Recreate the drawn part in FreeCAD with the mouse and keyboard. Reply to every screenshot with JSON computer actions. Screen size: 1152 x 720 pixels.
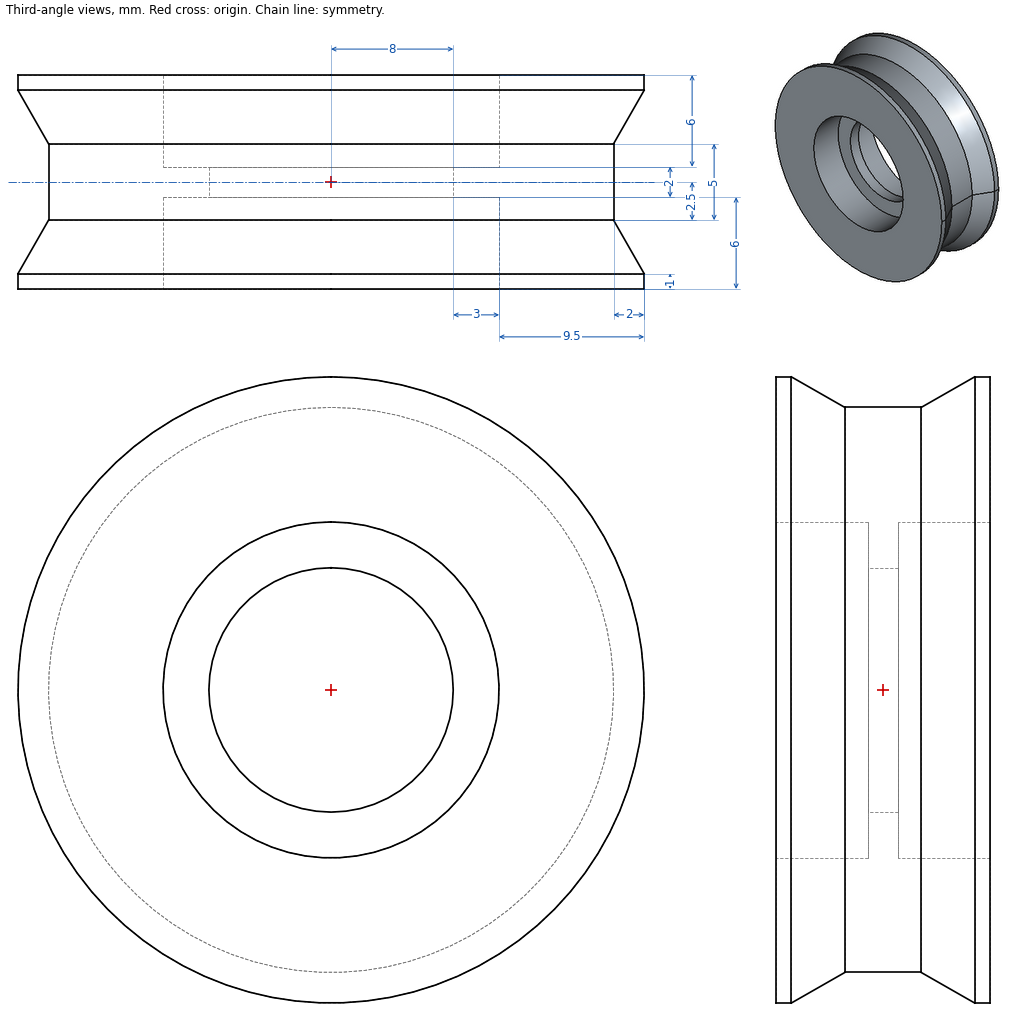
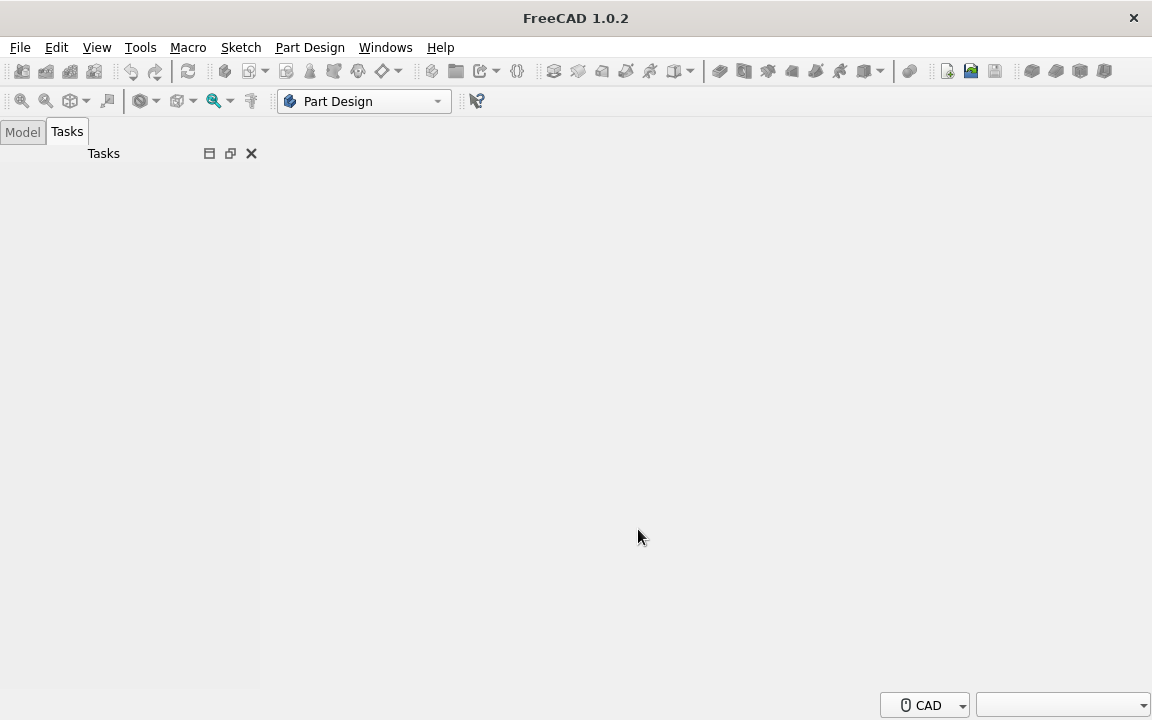
{"action": "left_click", "coordinate": [948, 72]}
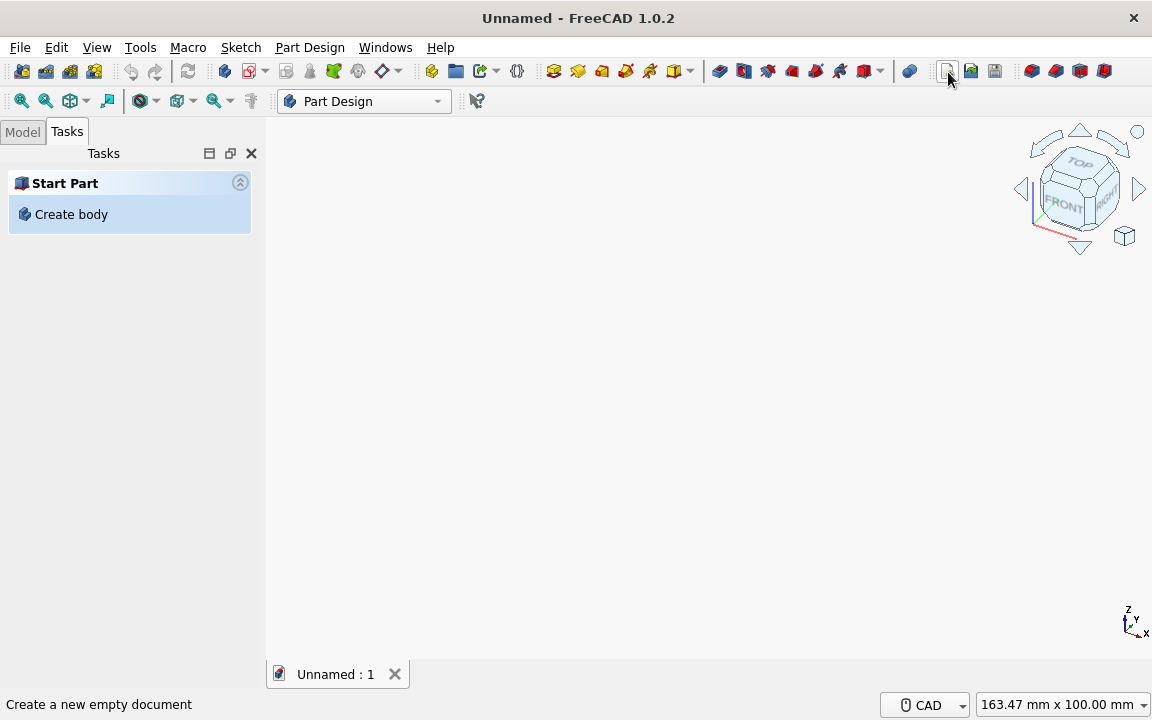
{"action": "left_click", "coordinate": [250, 72]}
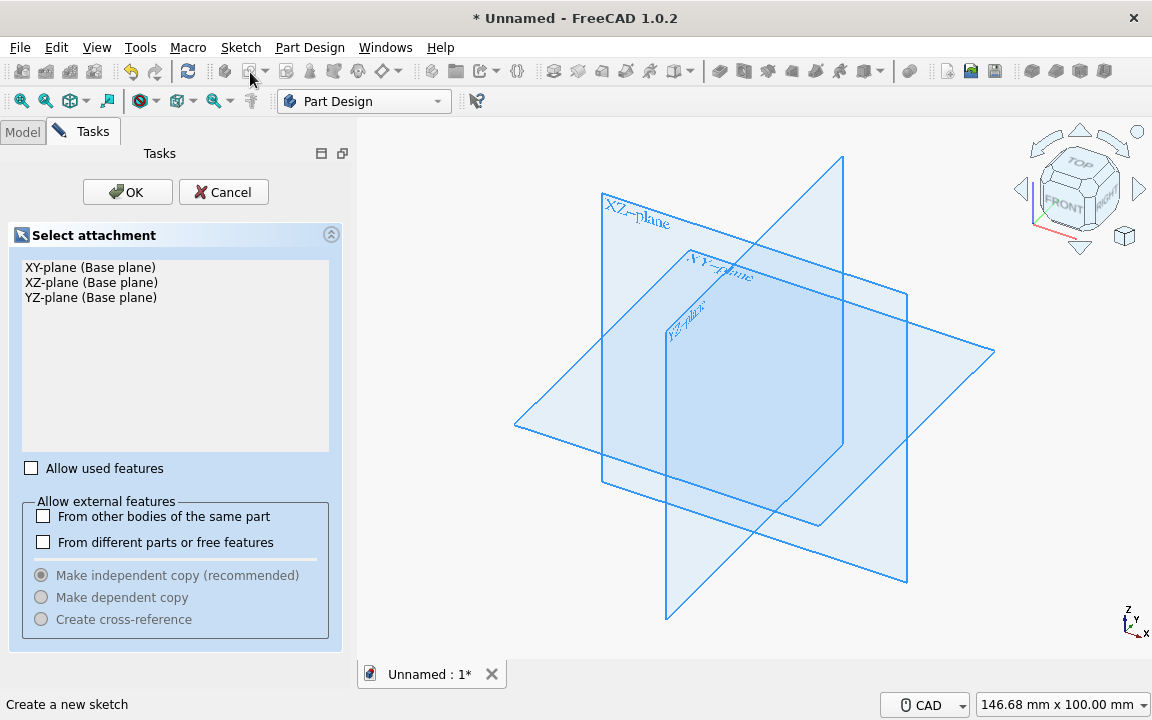
{"action": "left_click", "coordinate": [82, 268]}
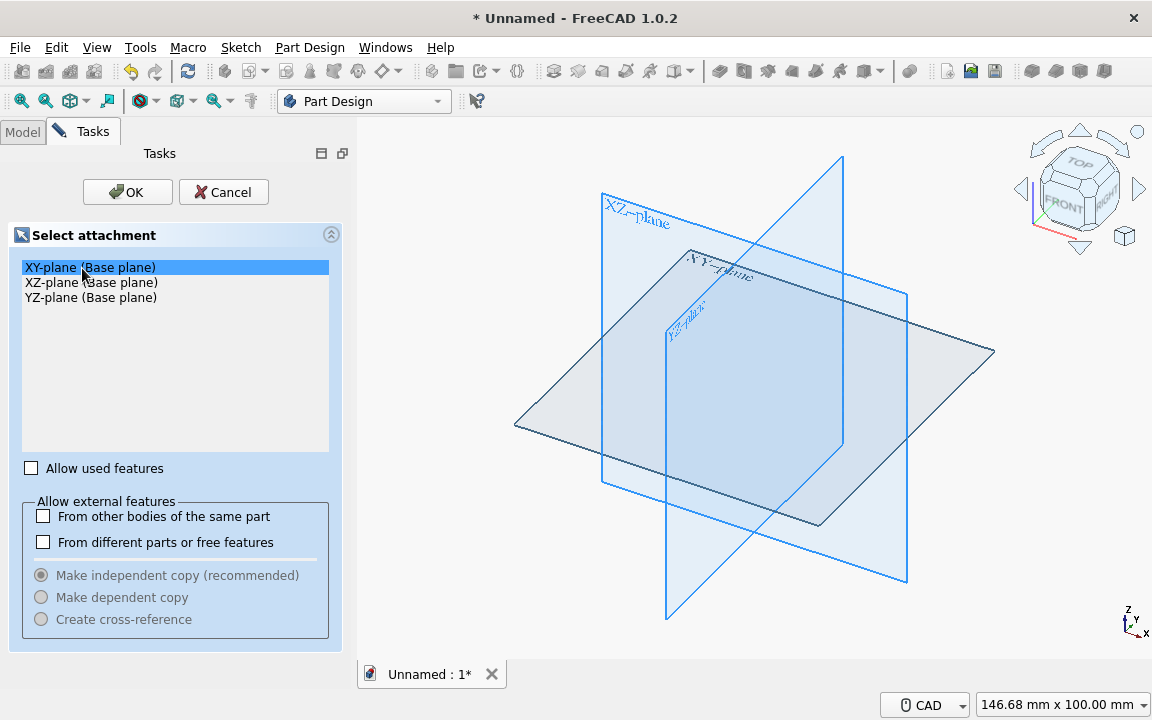
{"action": "left_click", "coordinate": [128, 192]}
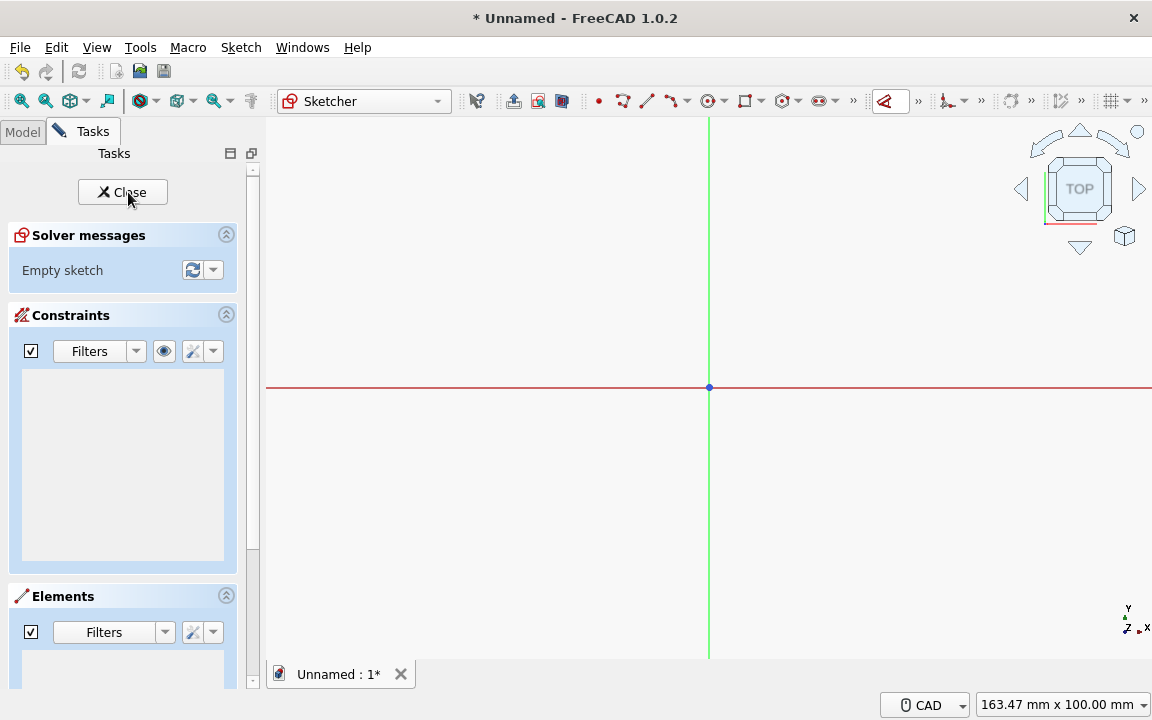
{"action": "scroll", "coordinate": [805, 388], "scroll_direction": "up", "scroll_amount": 7}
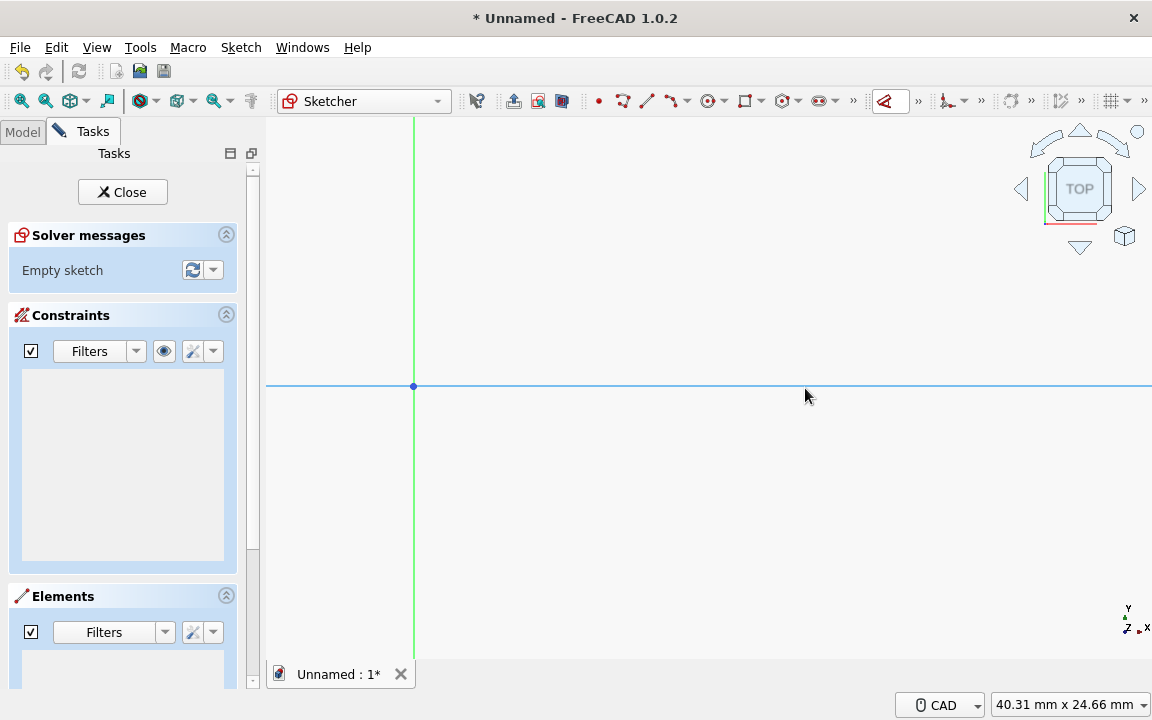
{"action": "left_click", "coordinate": [624, 102]}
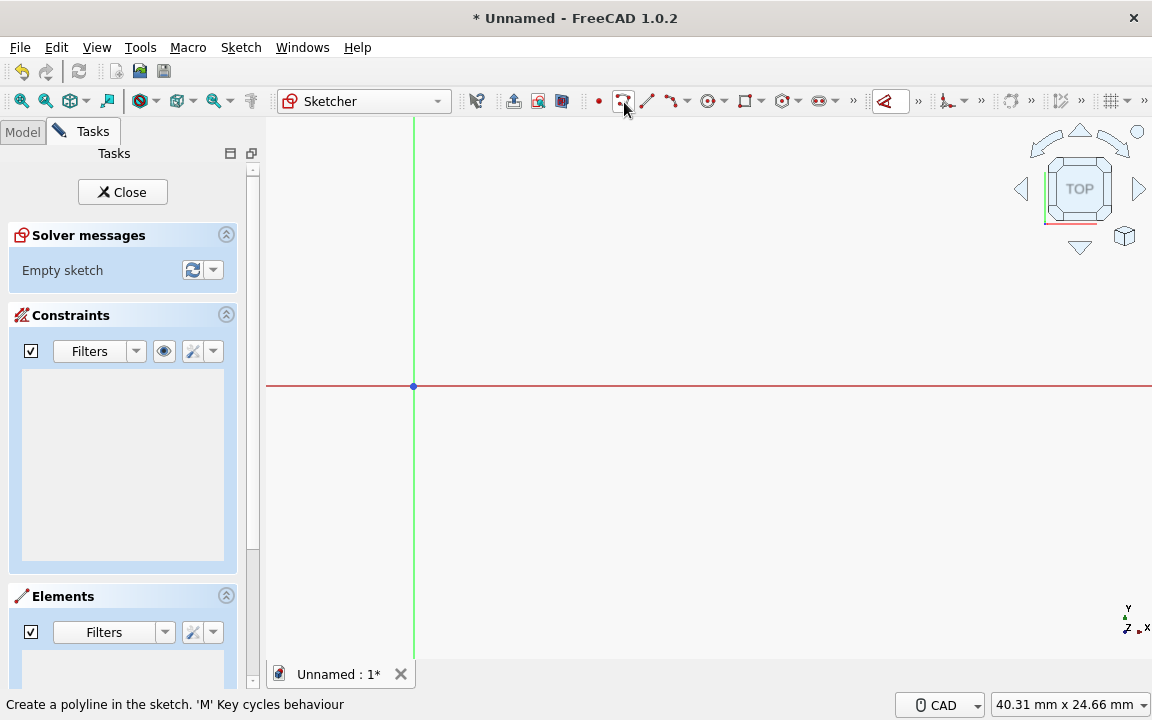
{"action": "left_click", "coordinate": [590, 364]}
{"action": "left_click", "coordinate": [590, 408]}
{"action": "left_click", "coordinate": [656, 408]}
{"action": "left_click", "coordinate": [656, 540]}
{"action": "left_click", "coordinate": [864, 540]}
{"action": "left_click", "coordinate": [864, 518]}
{"action": "left_click", "coordinate": [820, 441]}
{"action": "left_click", "coordinate": [820, 332]}
{"action": "left_click", "coordinate": [864, 255]}
{"action": "left_click", "coordinate": [864, 233]}
{"action": "left_click", "coordinate": [656, 233]}
{"action": "left_click", "coordinate": [656, 364]}
{"action": "left_click", "coordinate": [590, 365]}
{"action": "key", "text": "Escape"}
{"action": "key", "text": "Escape"}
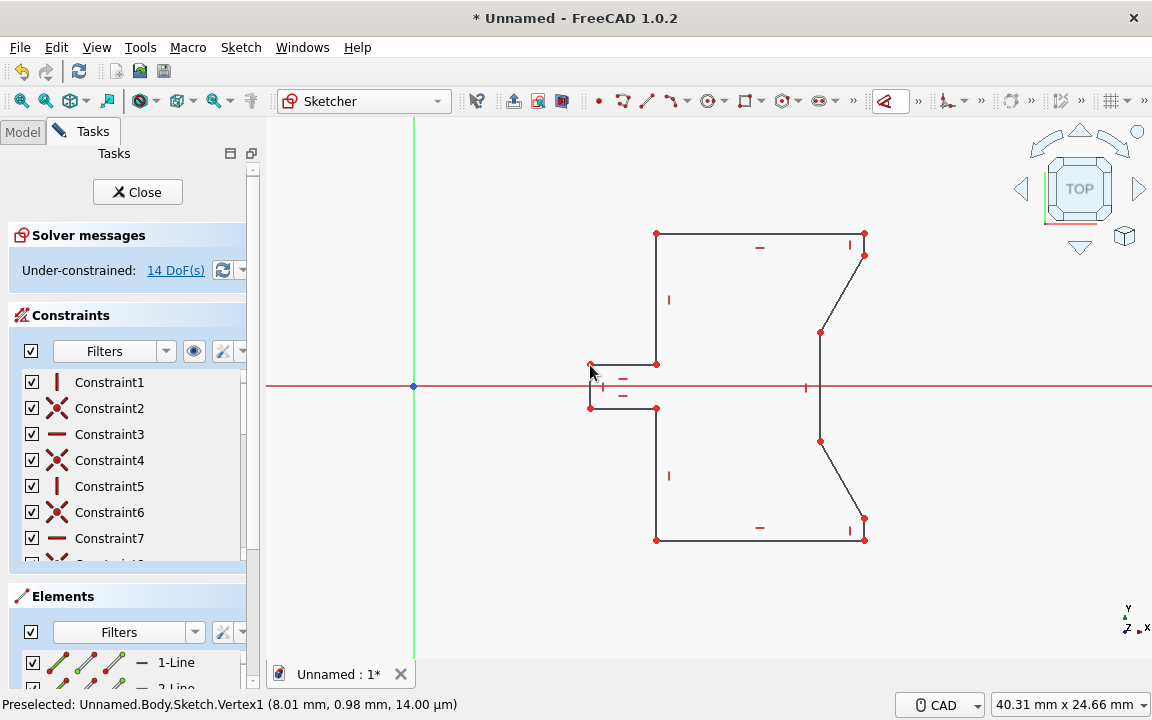
{"action": "left_click", "coordinate": [864, 519]}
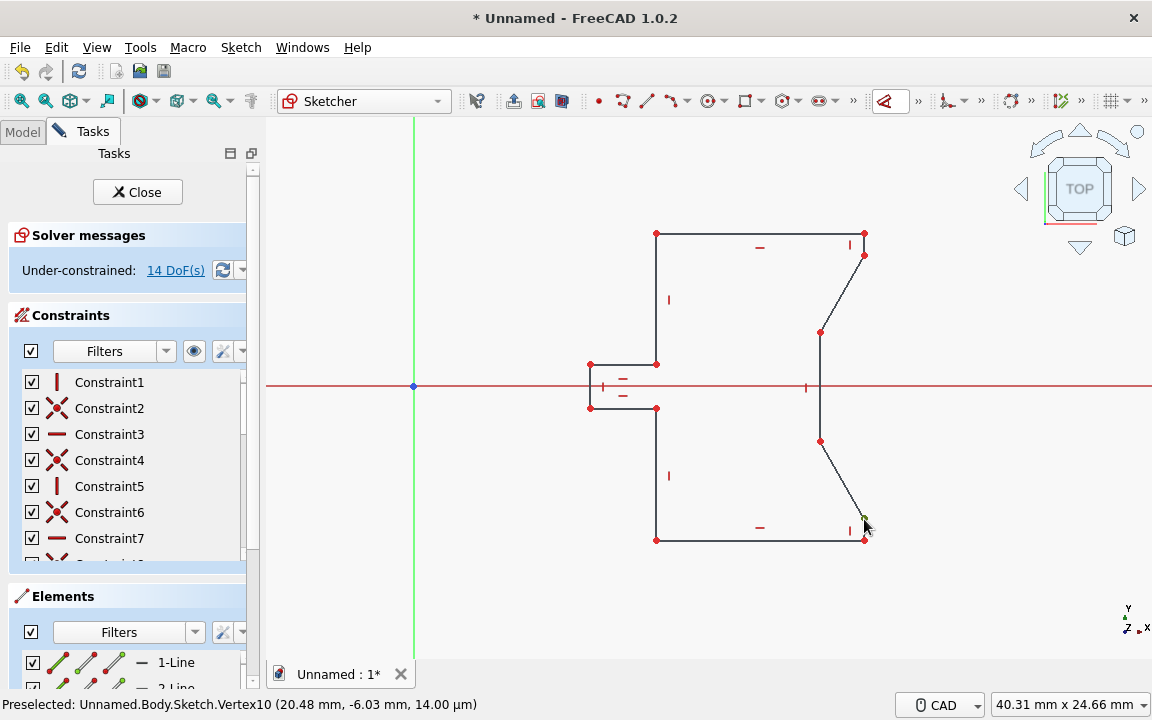
{"action": "left_click", "coordinate": [864, 256]}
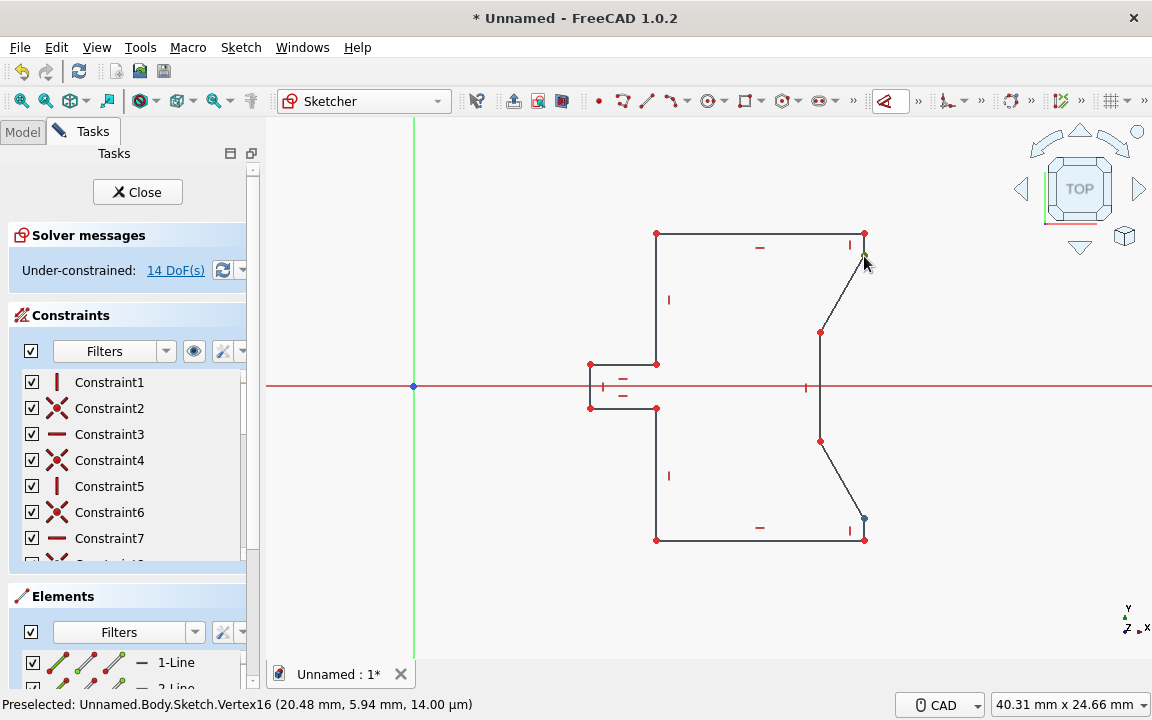
{"action": "left_click", "coordinate": [344, 386]}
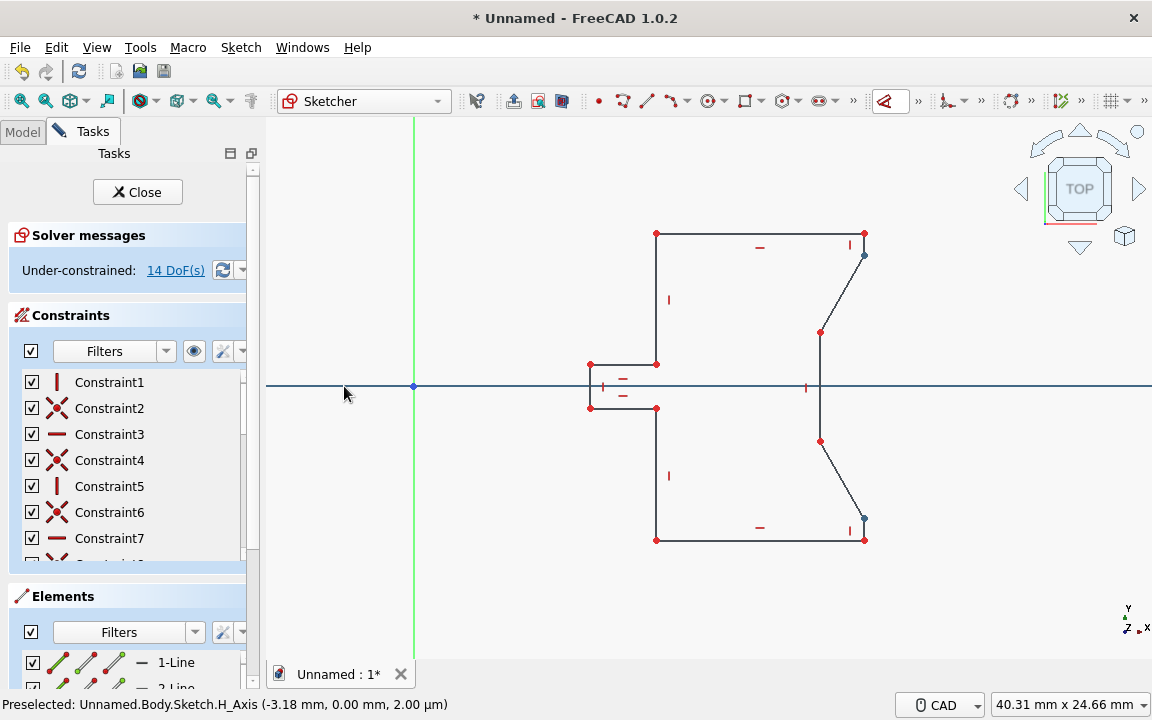
{"action": "key", "text": "s"}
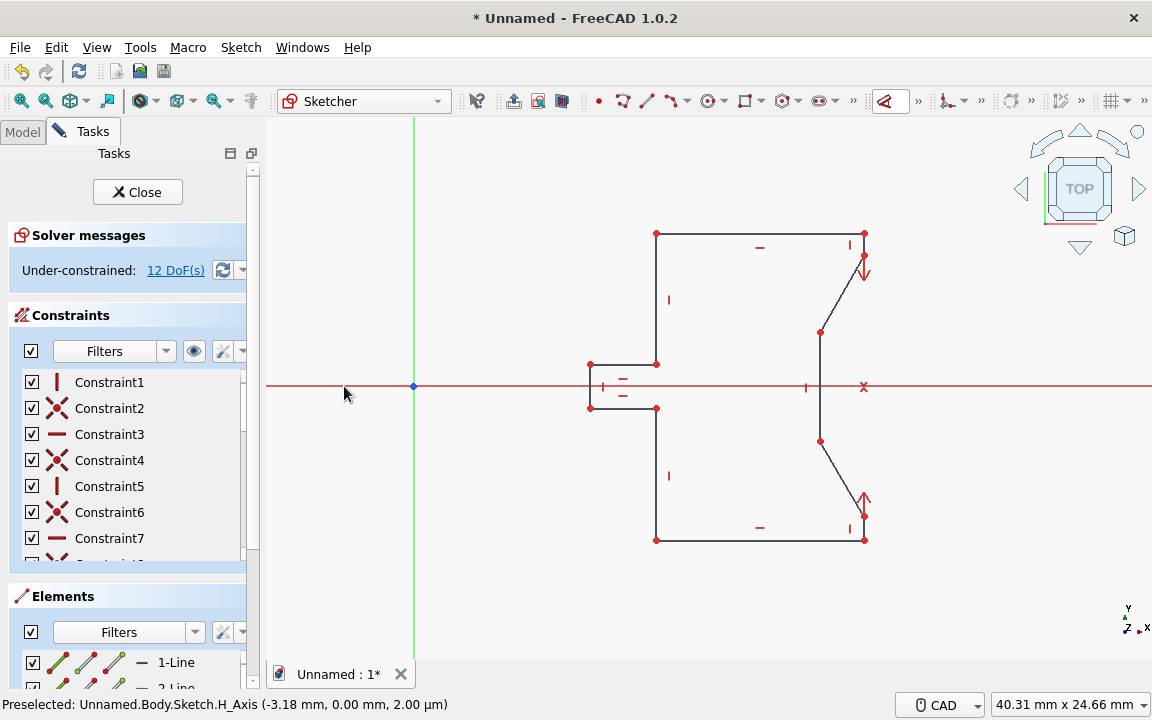
{"action": "left_click", "coordinate": [656, 541]}